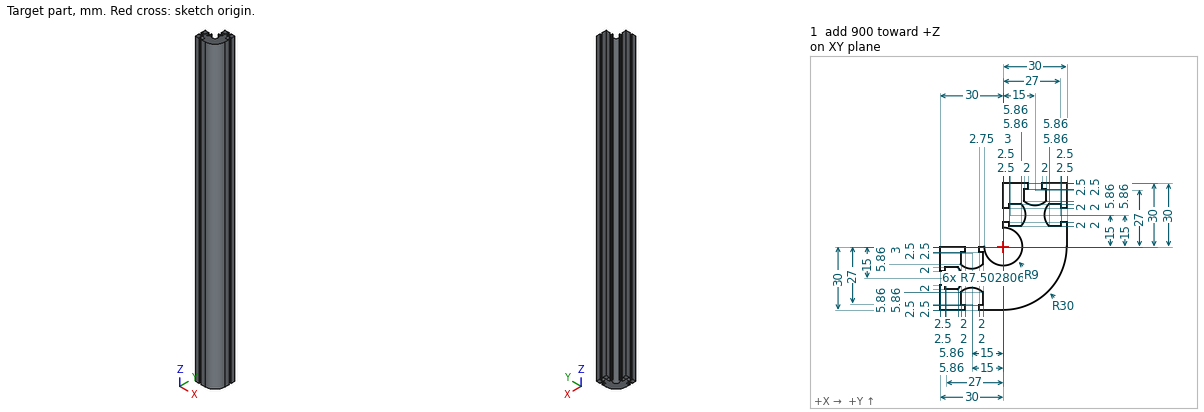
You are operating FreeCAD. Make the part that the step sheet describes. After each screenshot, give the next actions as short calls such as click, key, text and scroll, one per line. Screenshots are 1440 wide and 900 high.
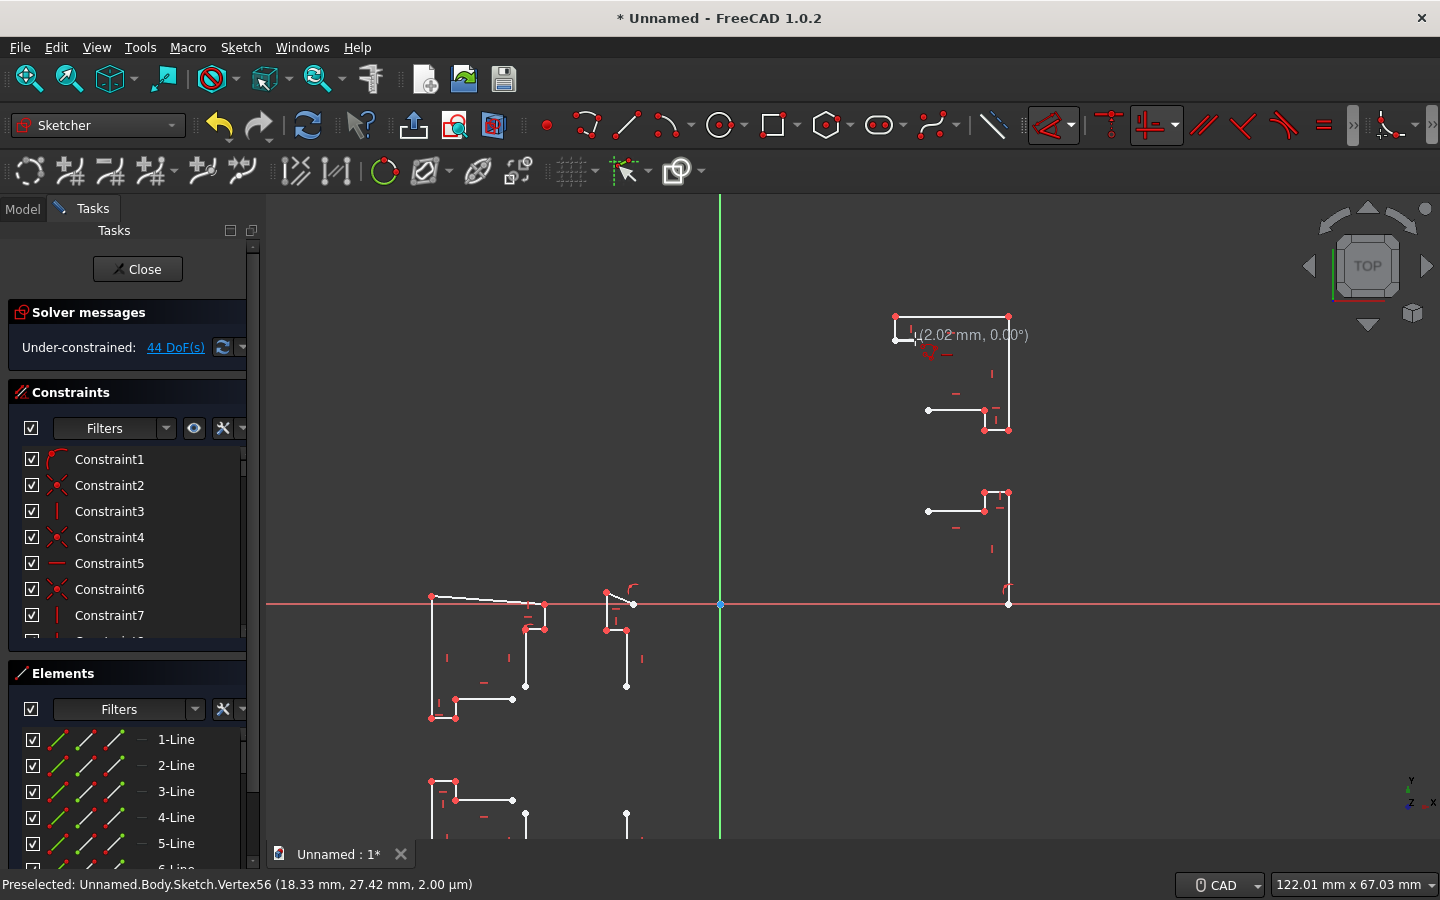
click(915, 339)
click(915, 396)
right_click(915, 396)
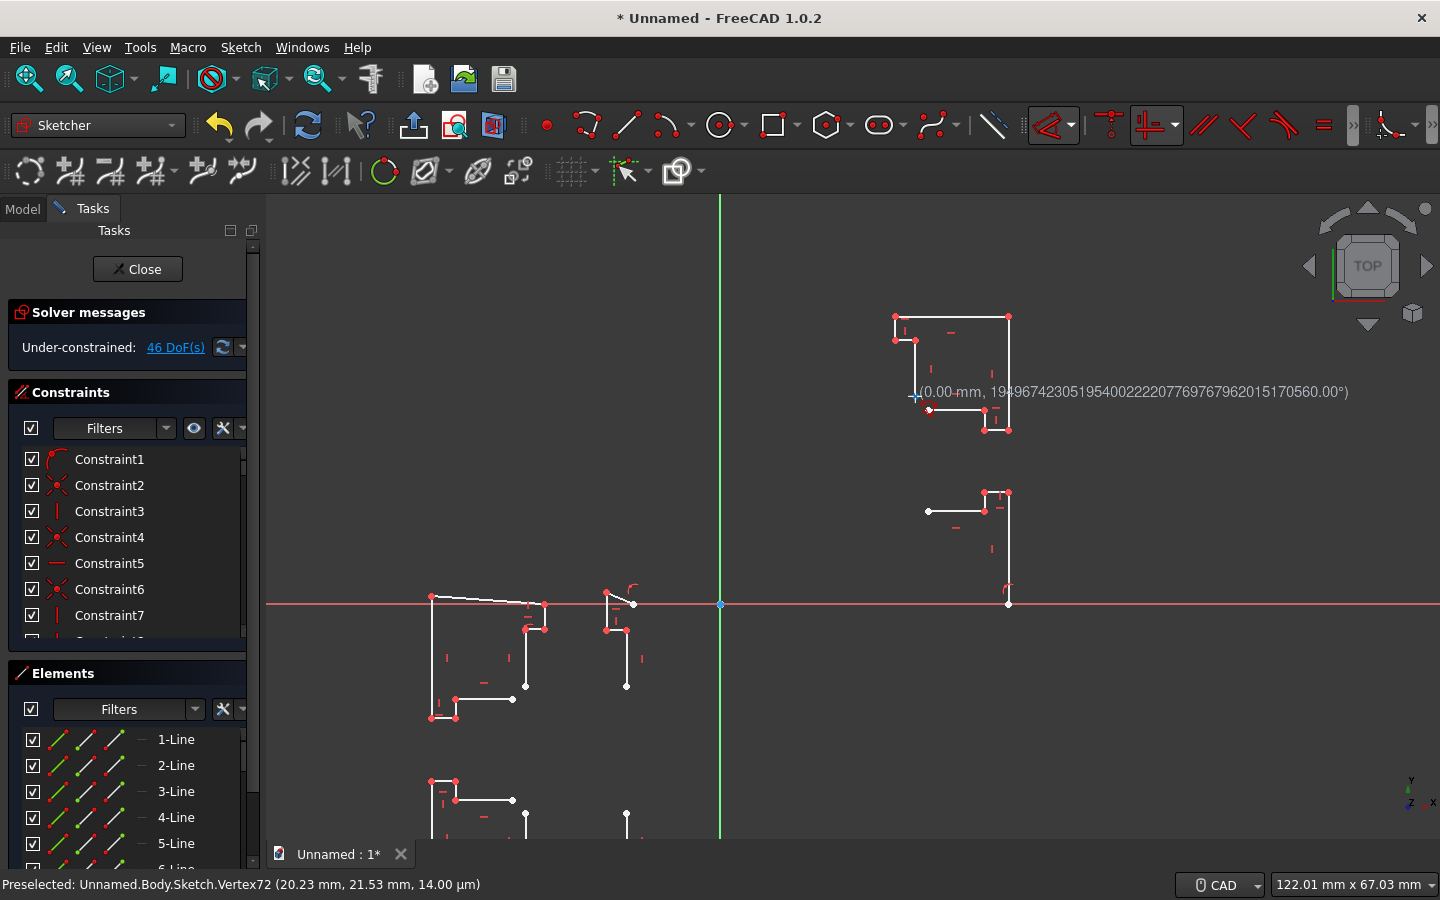
click(814, 396)
click(814, 340)
click(833, 340)
click(833, 316)
click(720, 316)
click(729, 429)
click(744, 429)
click(744, 409)
click(801, 409)
right_click(801, 409)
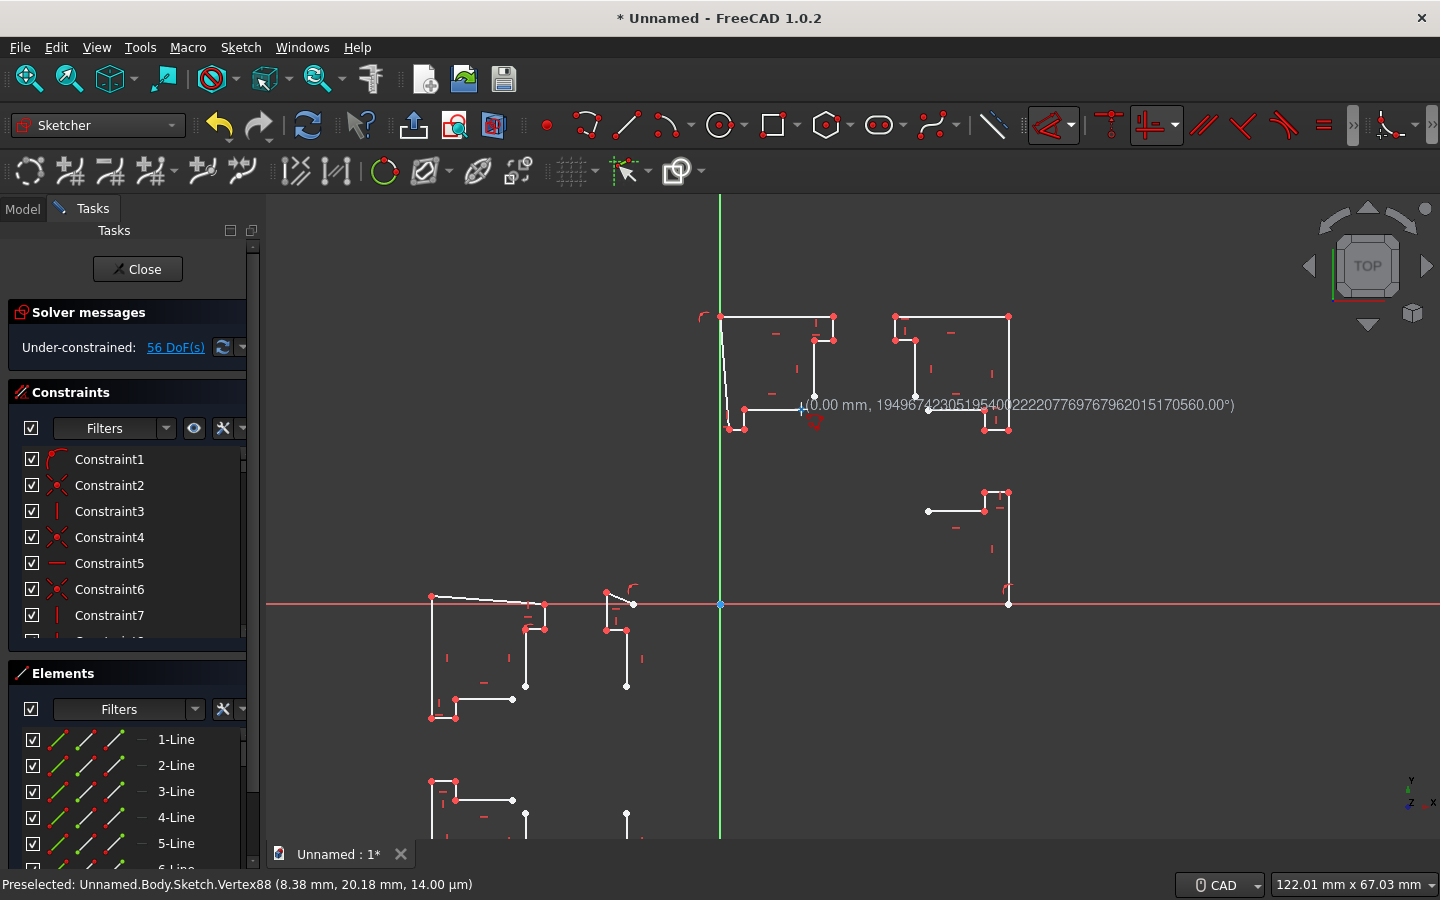
click(801, 510)
click(744, 510)
click(744, 491)
click(720, 491)
click(729, 518)
right_click(729, 518)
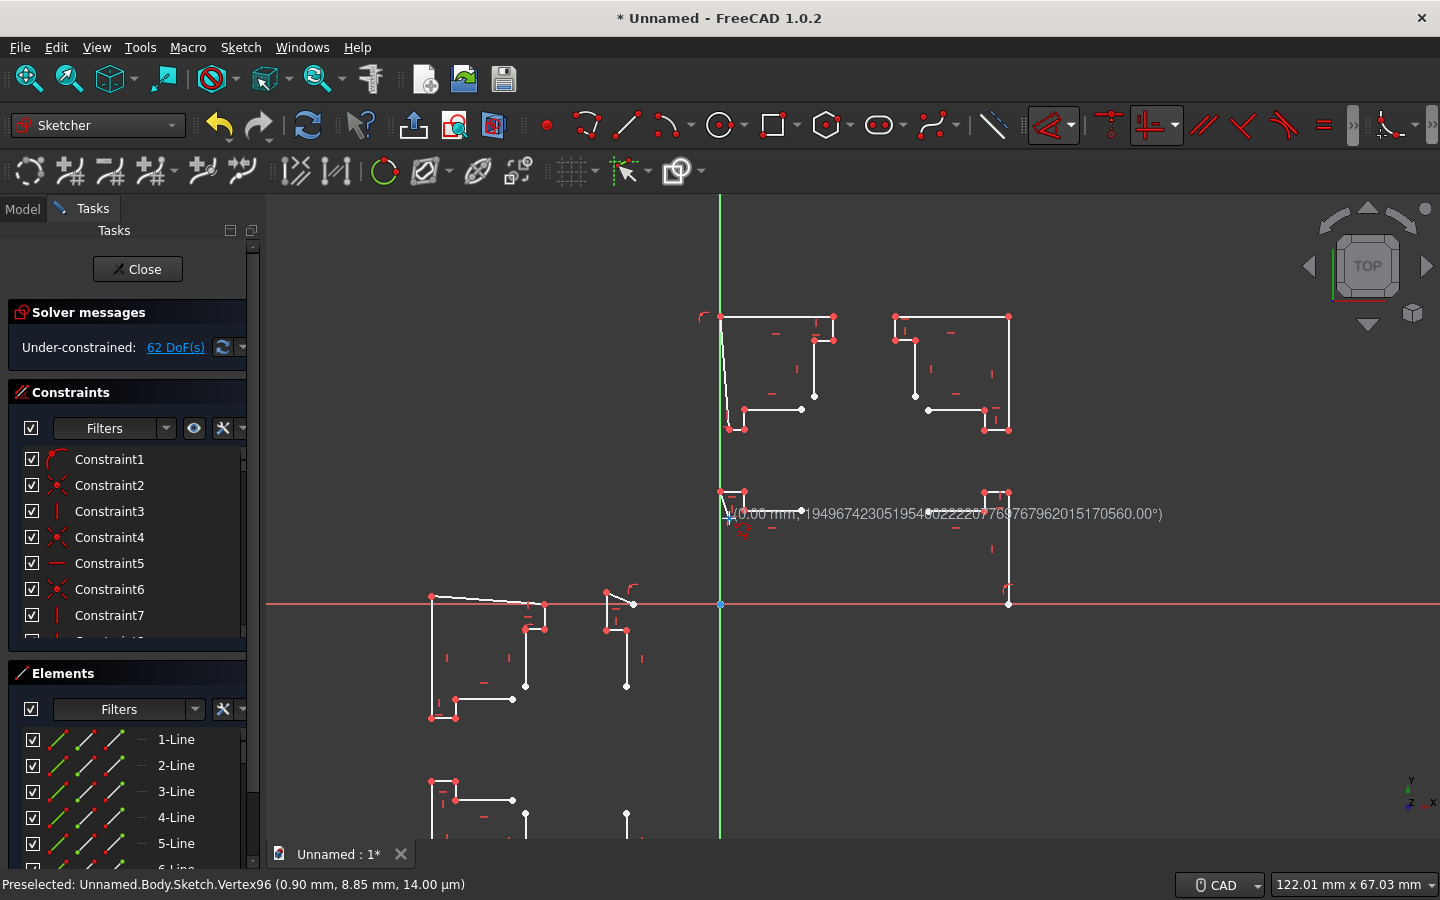
key(g)
key(3)
key(a)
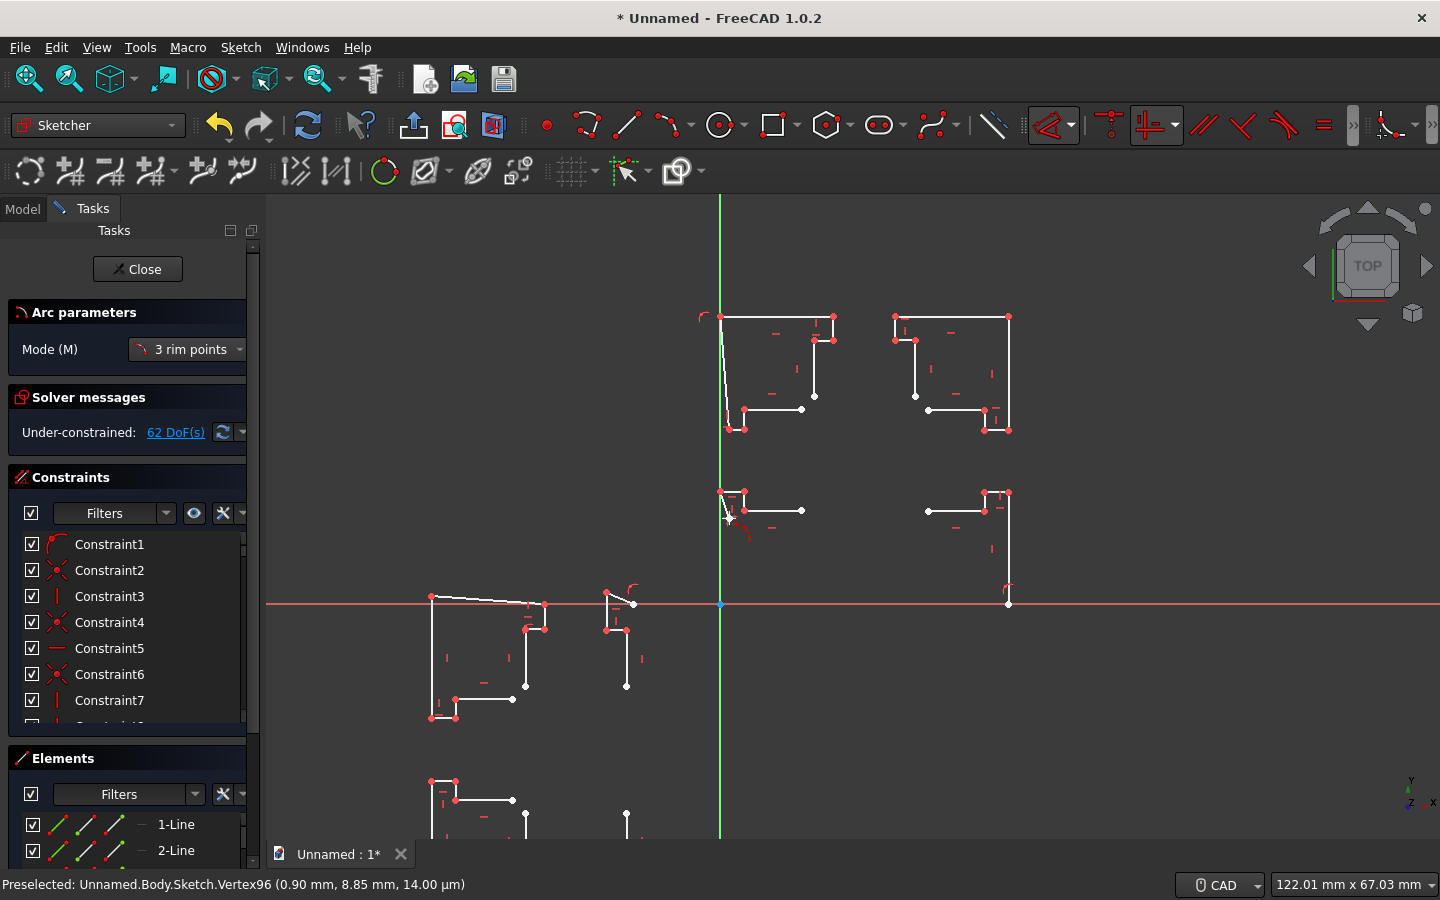
click(627, 686)
click(526, 686)
click(576, 705)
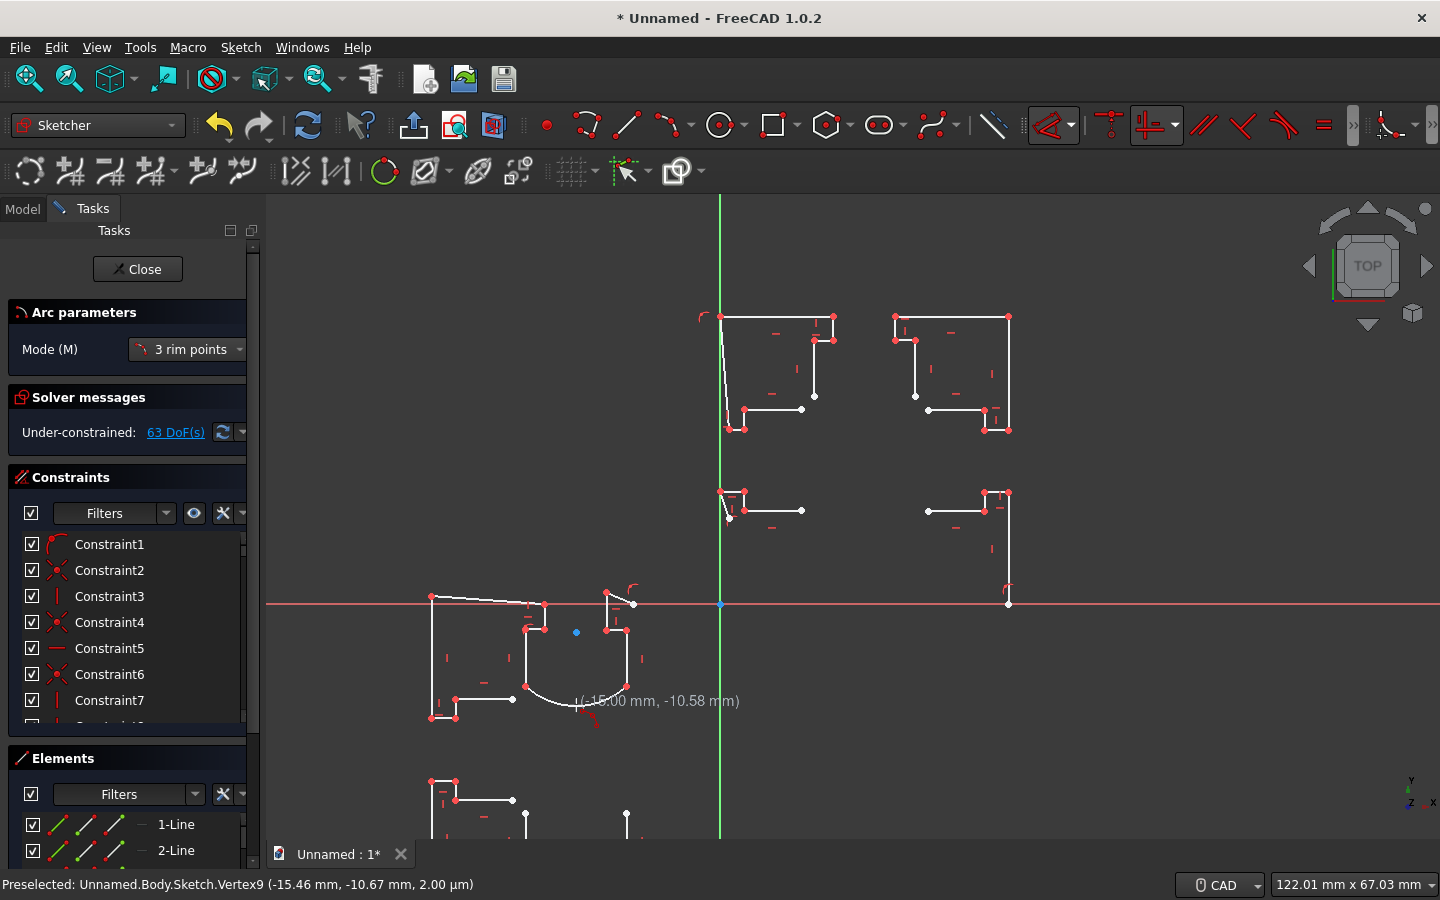
click(513, 699)
click(513, 800)
click(533, 749)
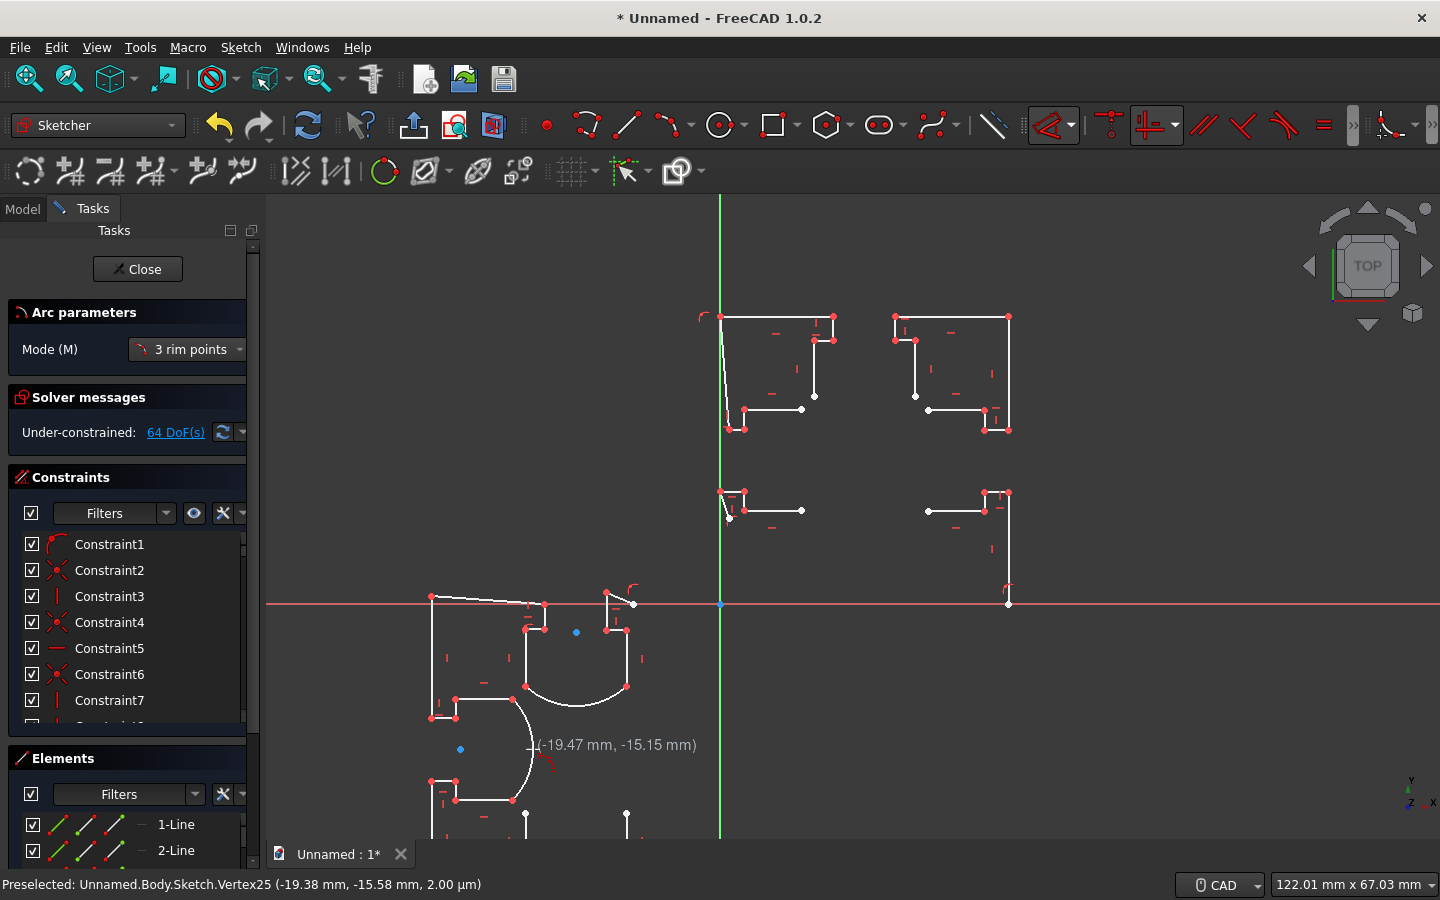
scroll(915, 338, down, 2)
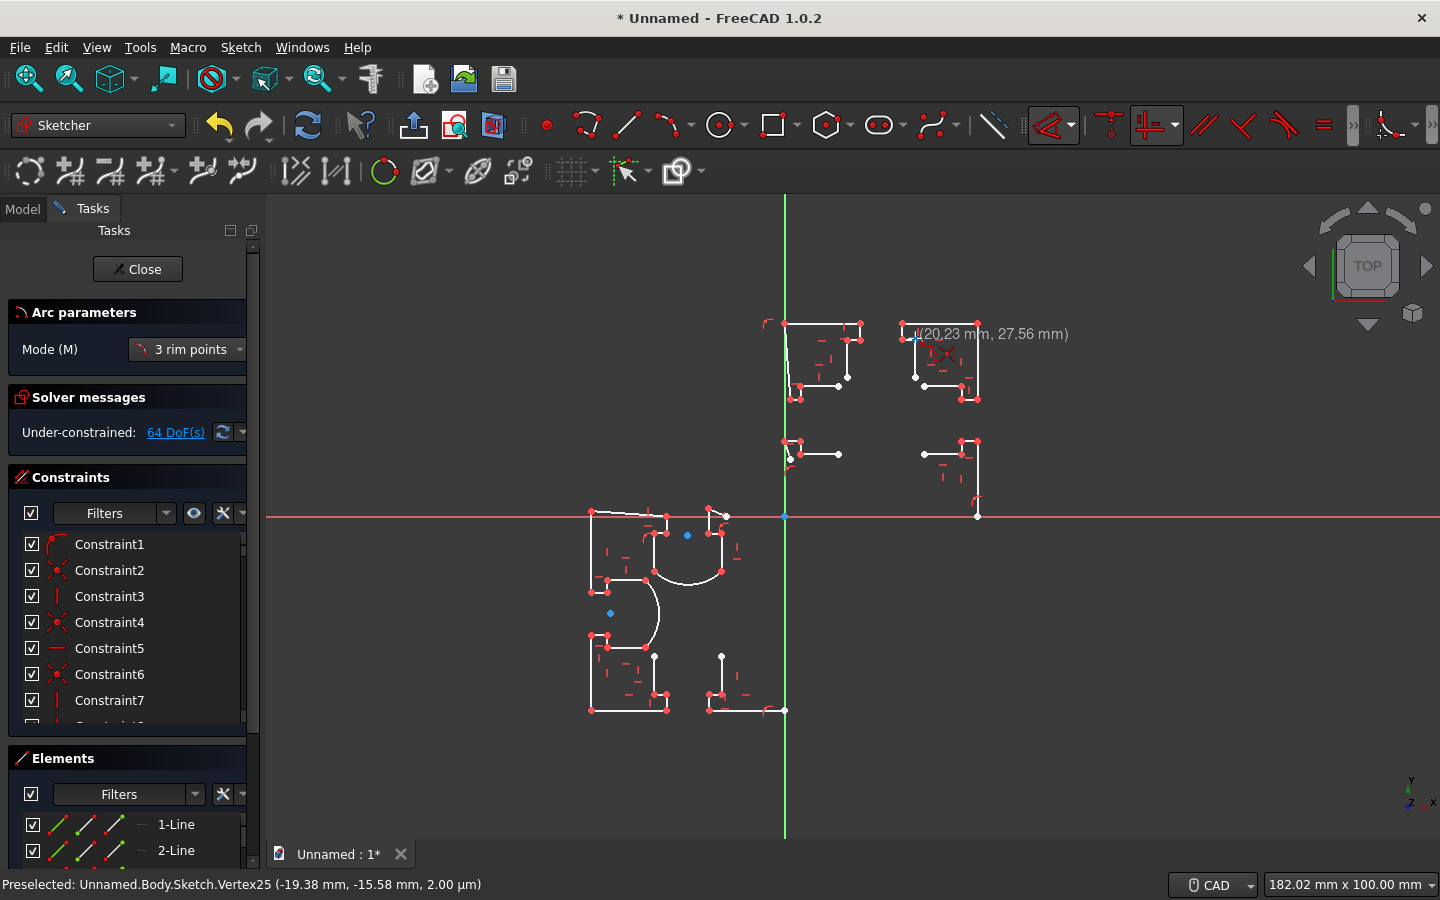
scroll(654, 656, up, 2)